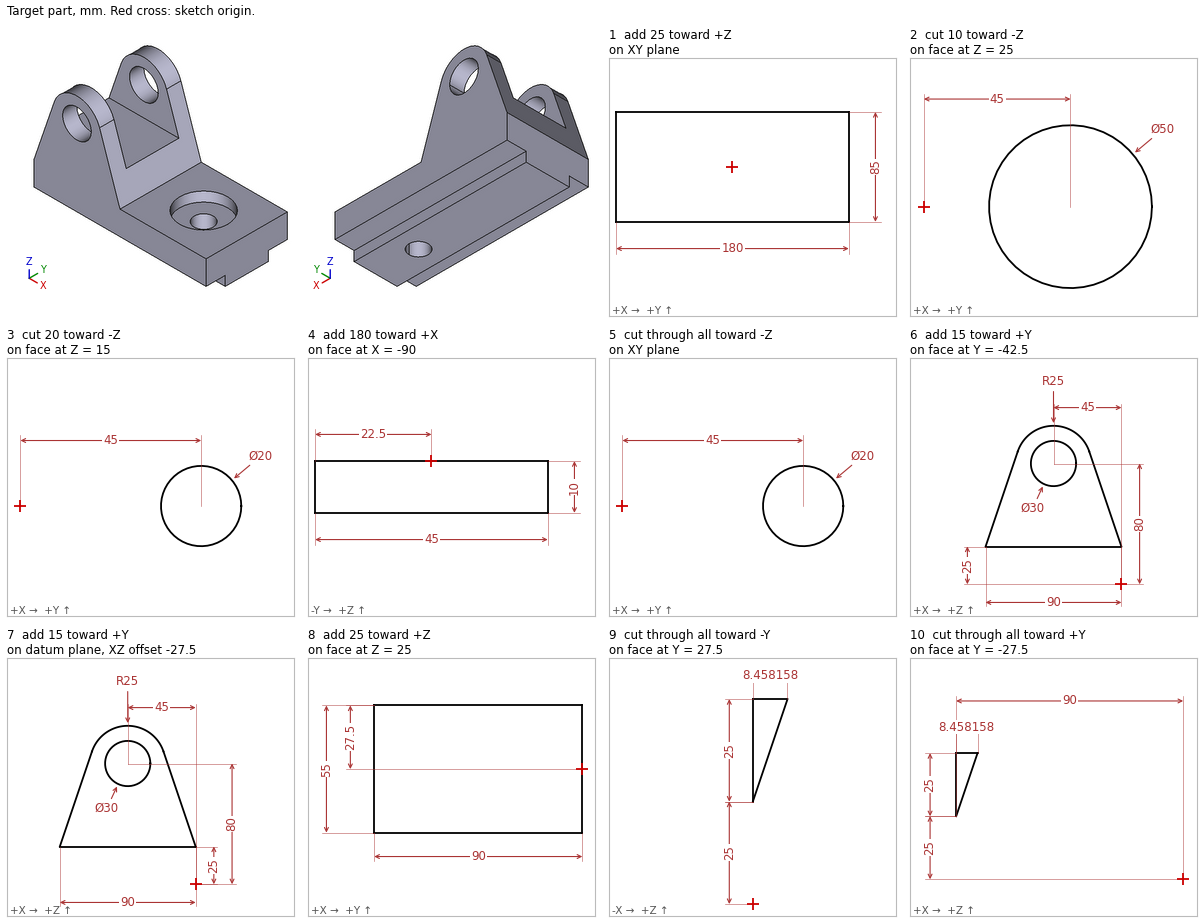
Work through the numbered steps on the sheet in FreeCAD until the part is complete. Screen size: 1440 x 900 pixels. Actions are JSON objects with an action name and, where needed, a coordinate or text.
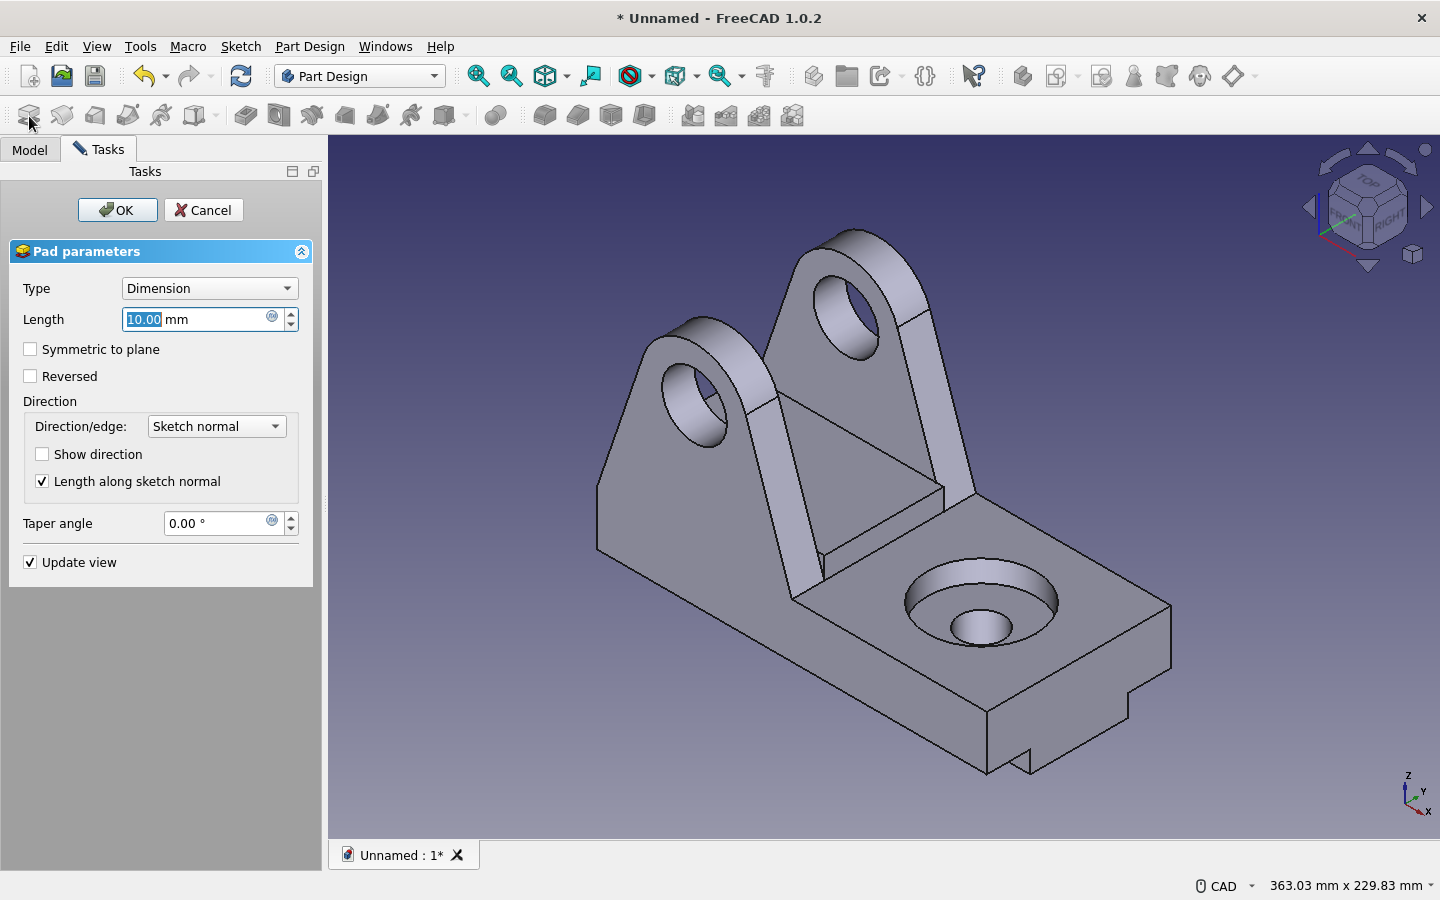
{"action": "type", "text": "25"}
{"action": "key", "text": "Tab"}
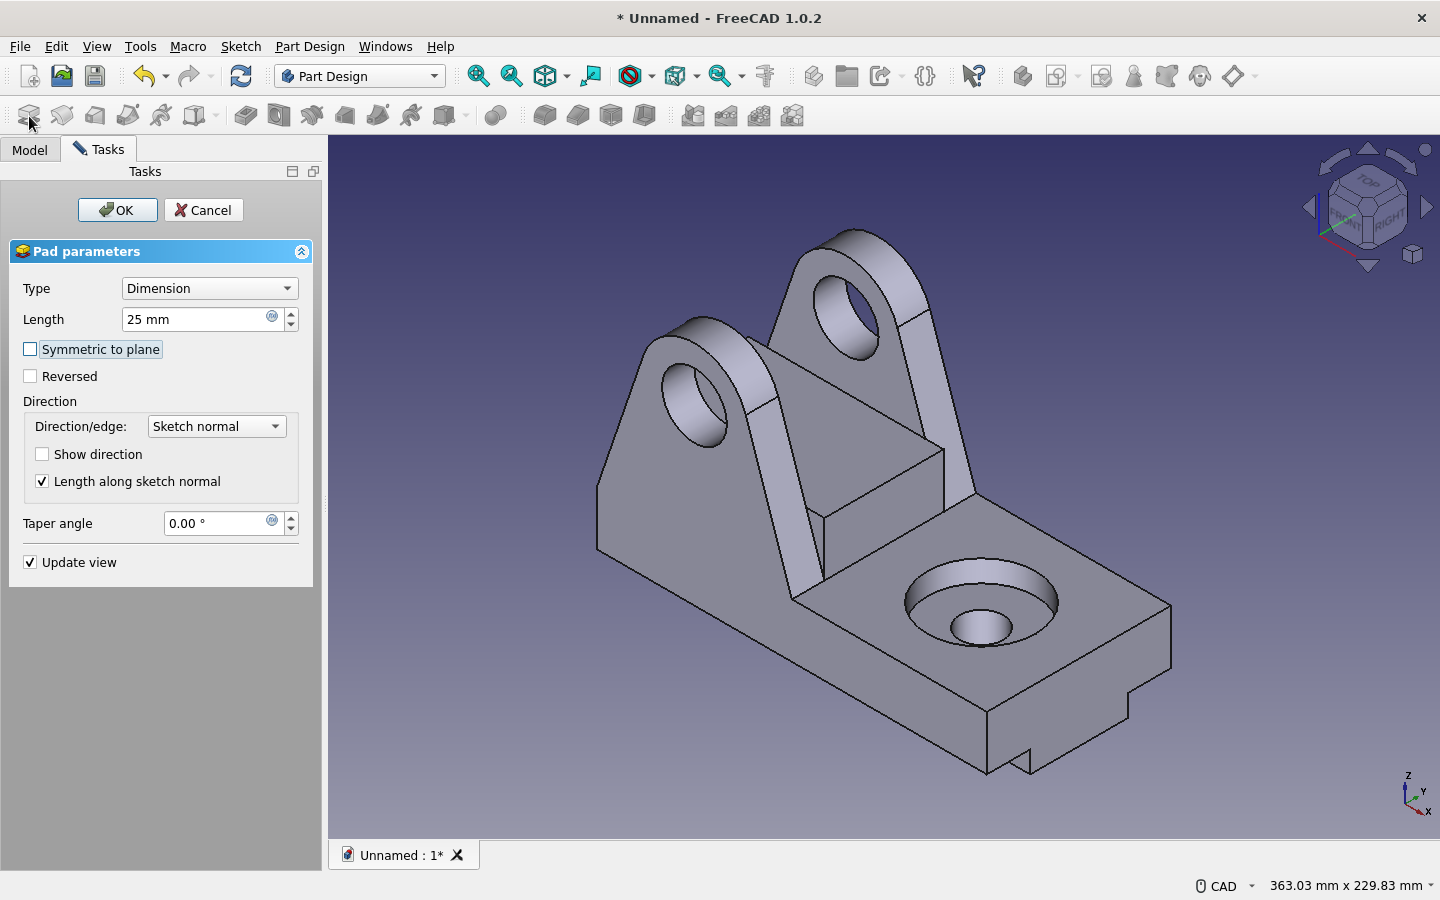
{"action": "left_click", "coordinate": [118, 210]}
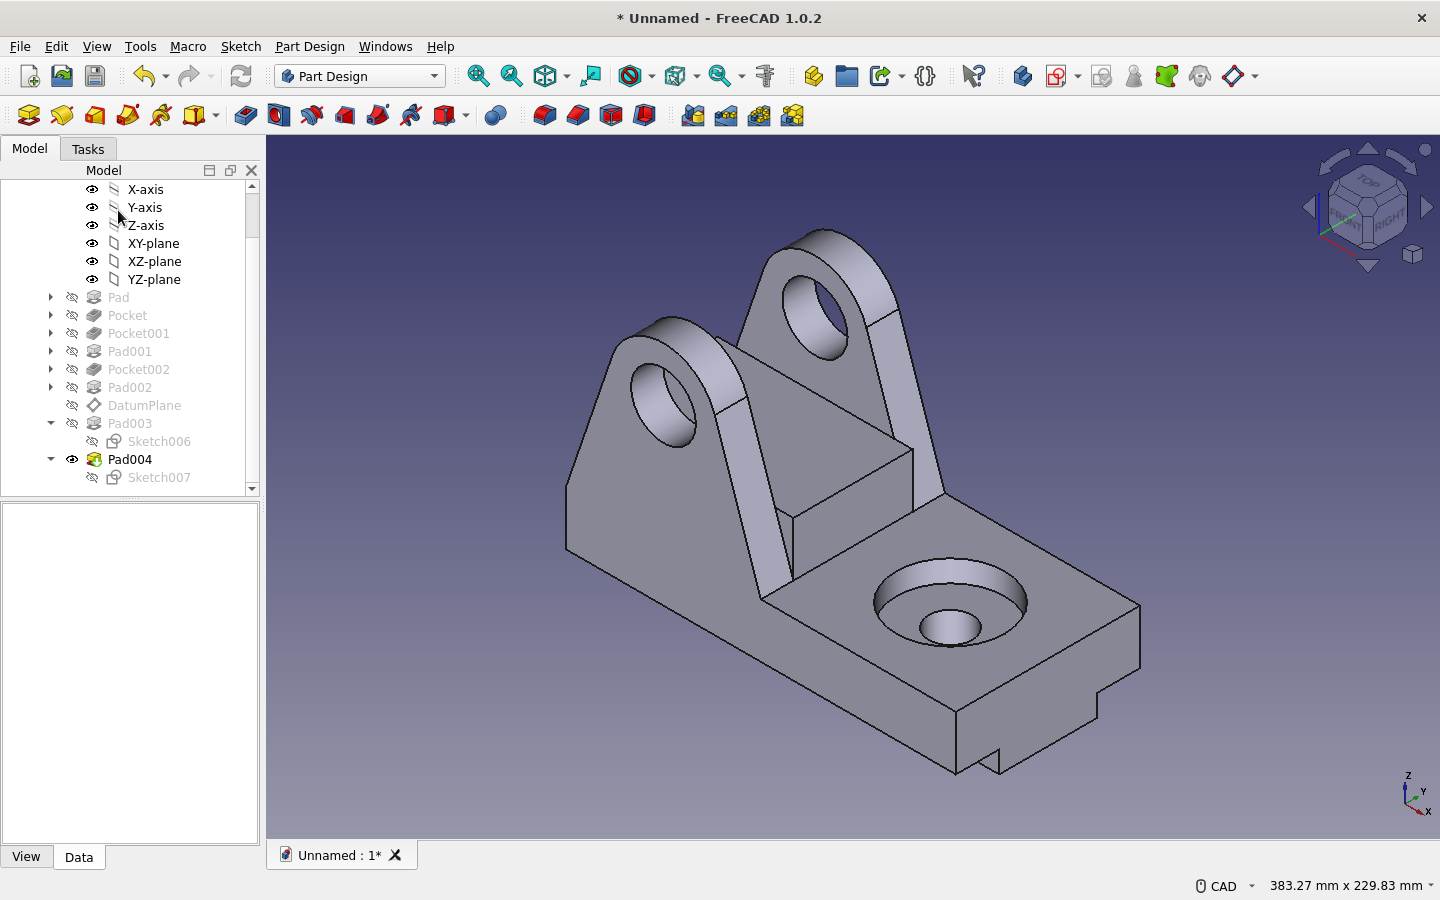
{"action": "key", "text": "4"}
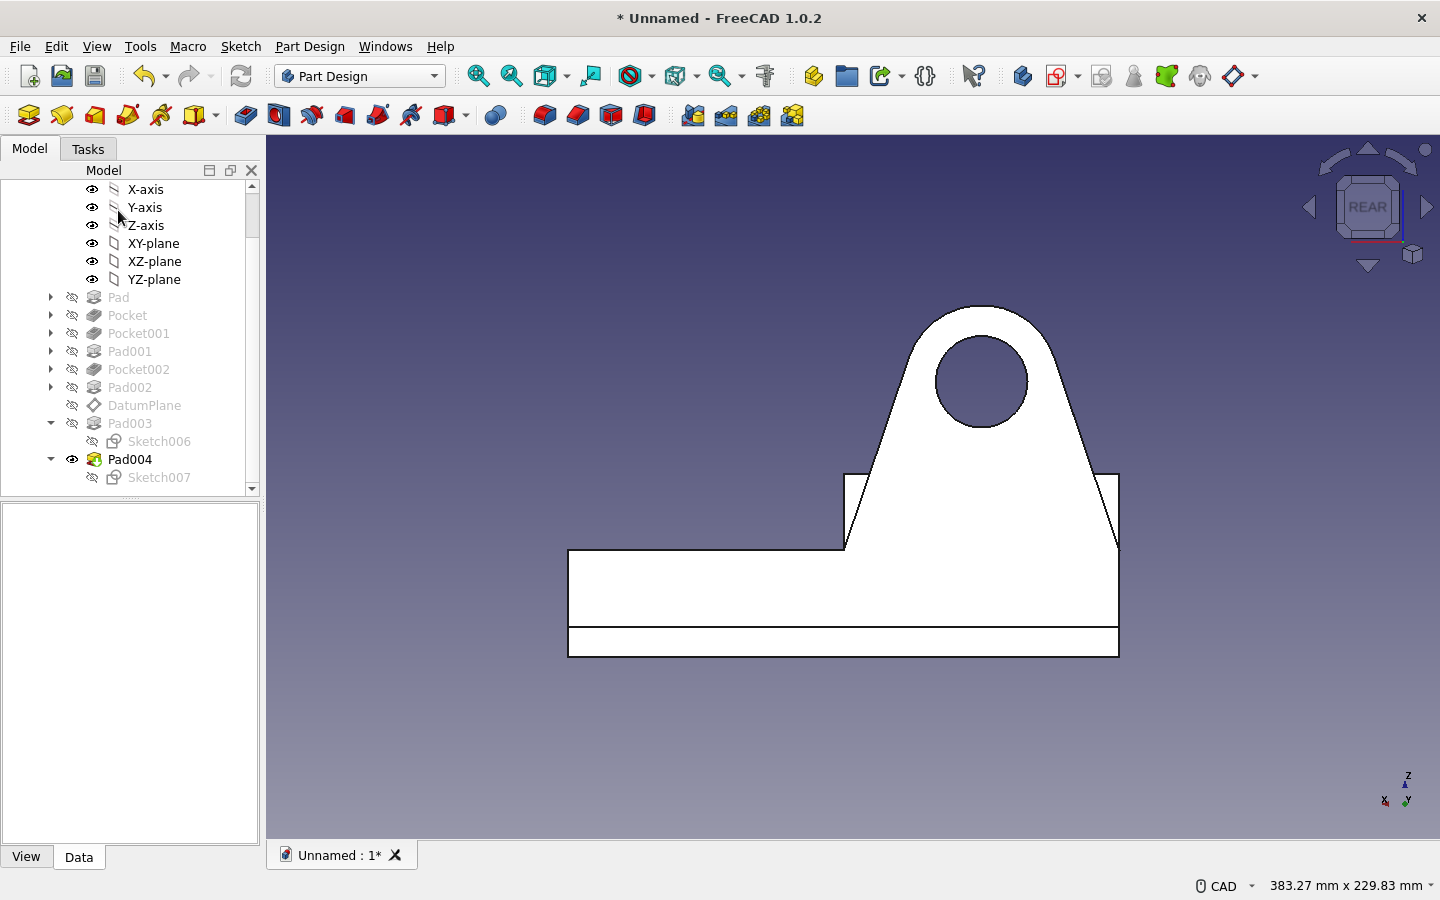
{"action": "left_click", "coordinate": [1110, 489]}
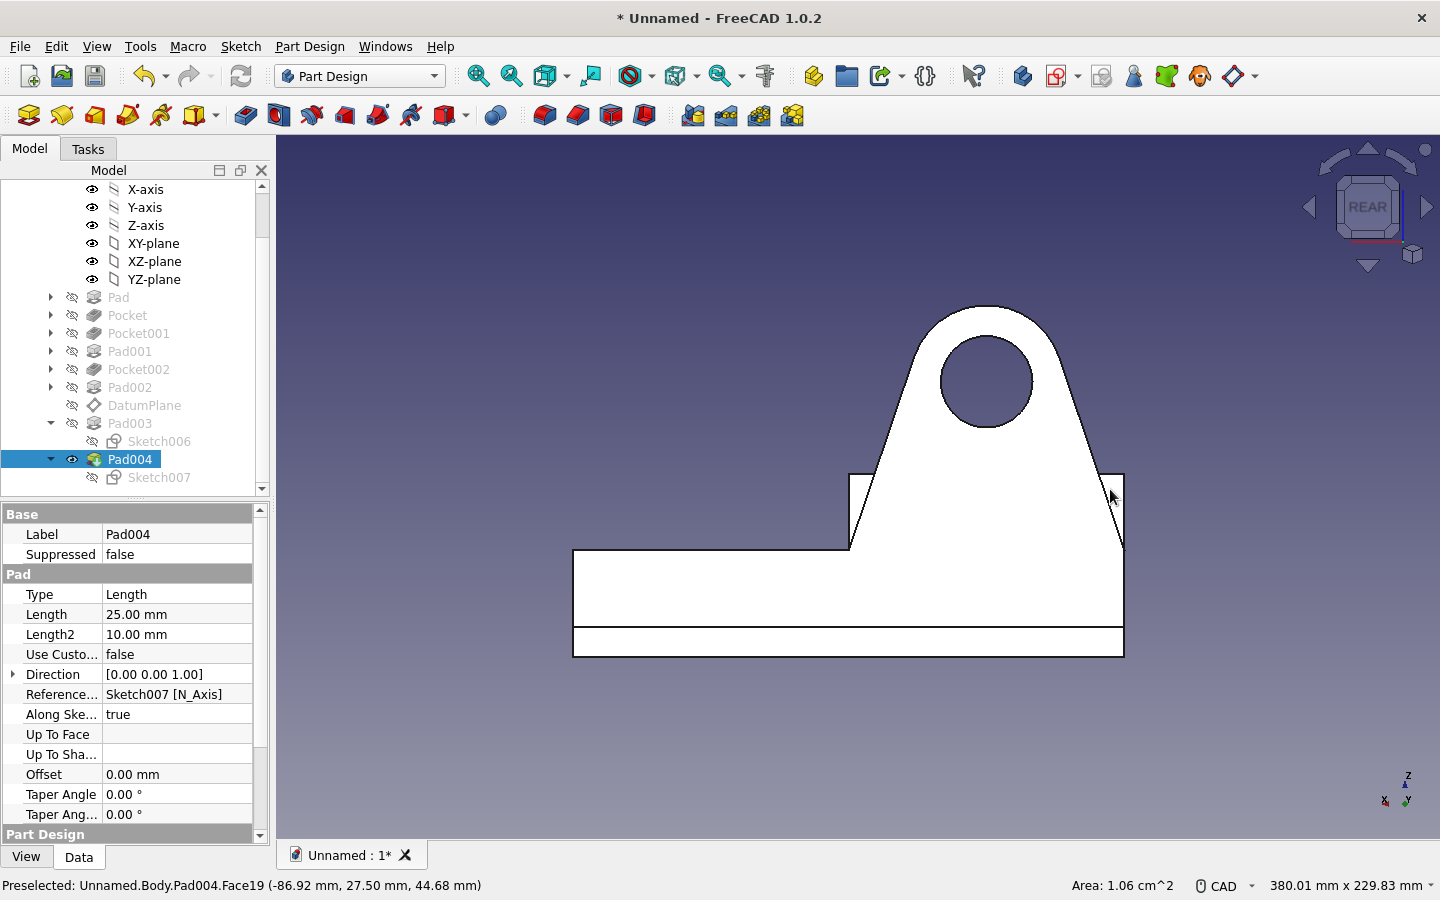
{"action": "left_click", "coordinate": [1056, 76]}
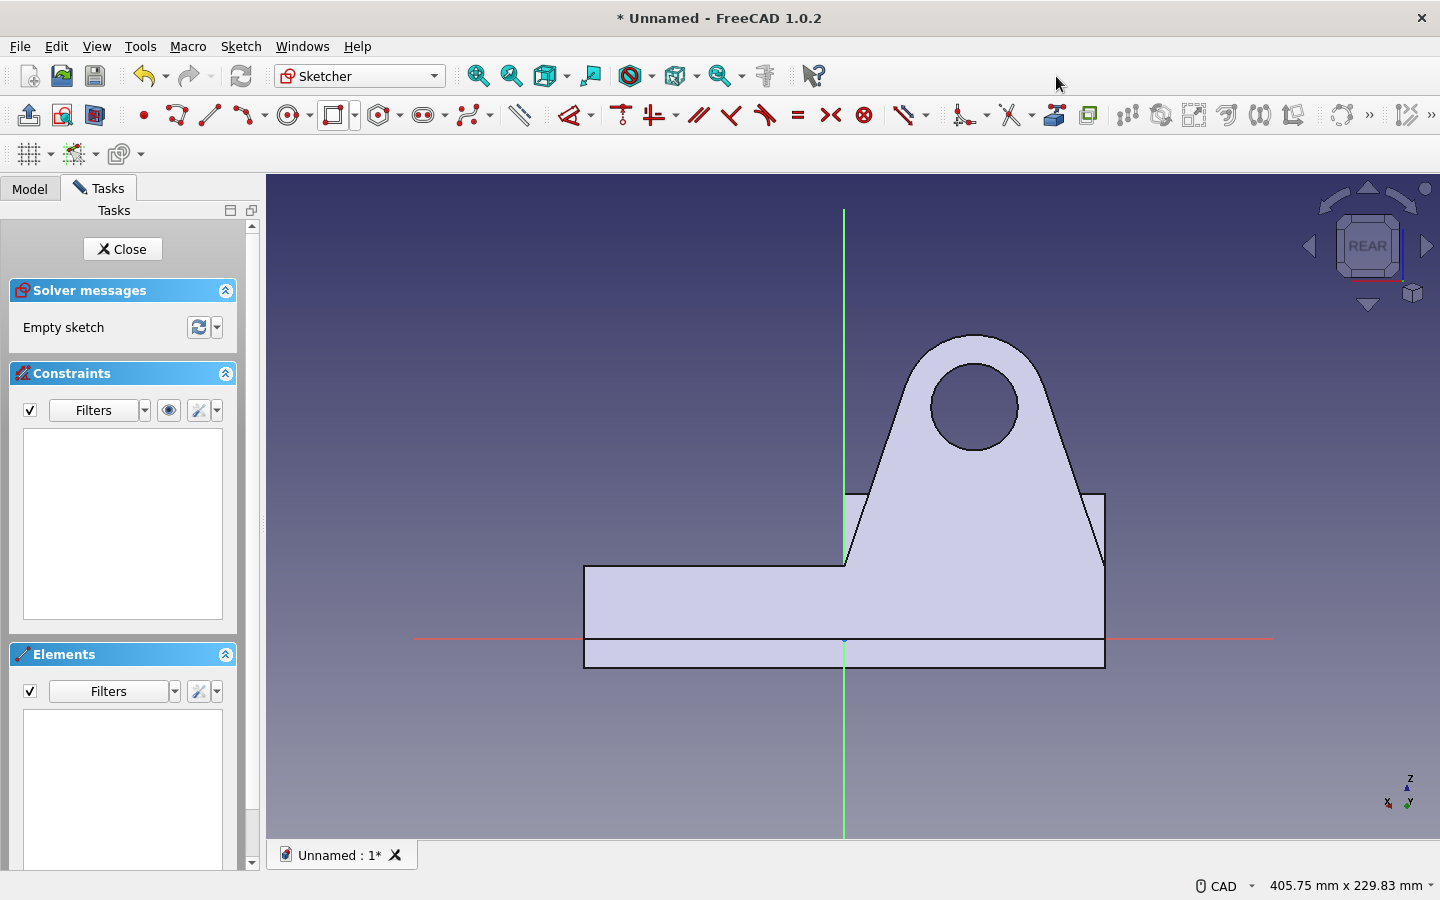
{"action": "scroll", "coordinate": [898, 601], "scroll_direction": "up", "scroll_amount": 5}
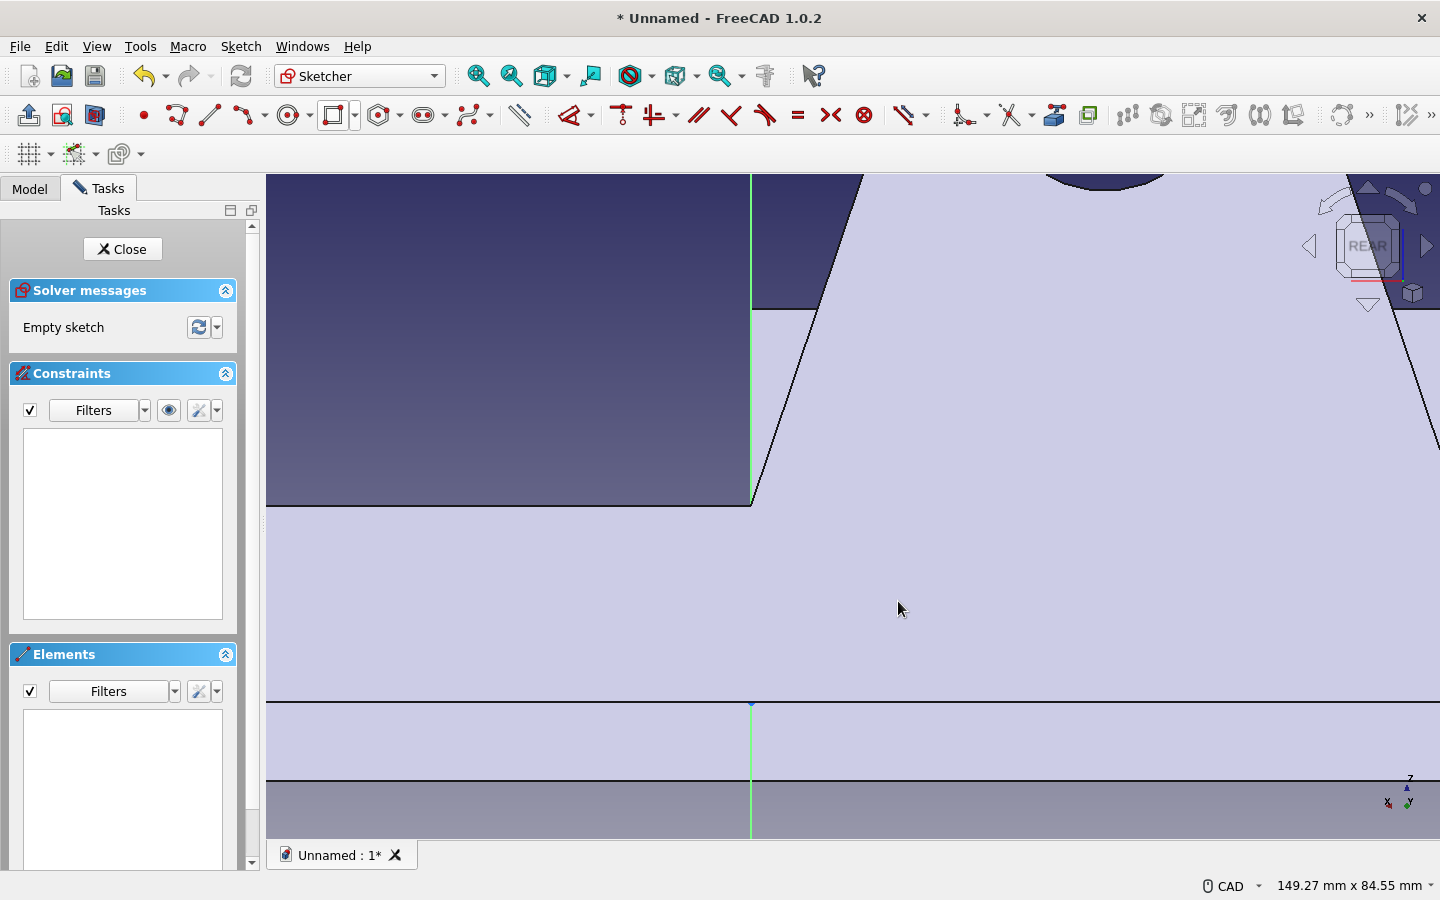
{"action": "left_click", "coordinate": [177, 116]}